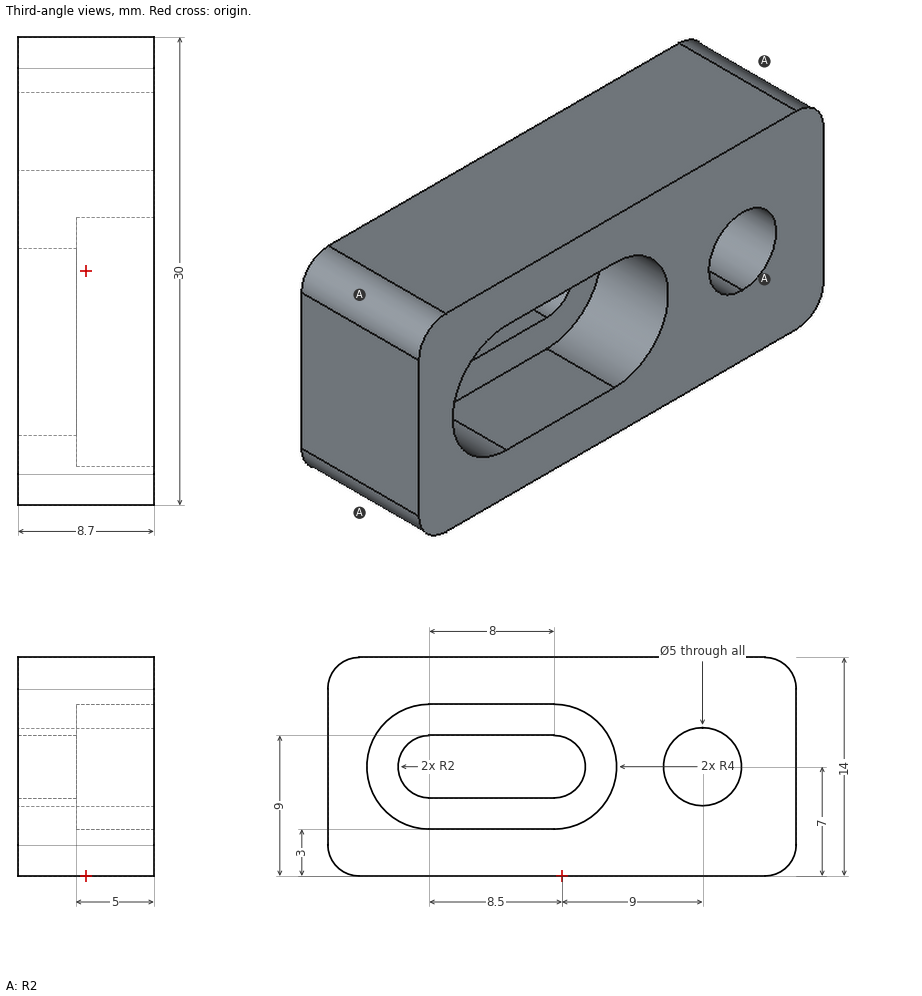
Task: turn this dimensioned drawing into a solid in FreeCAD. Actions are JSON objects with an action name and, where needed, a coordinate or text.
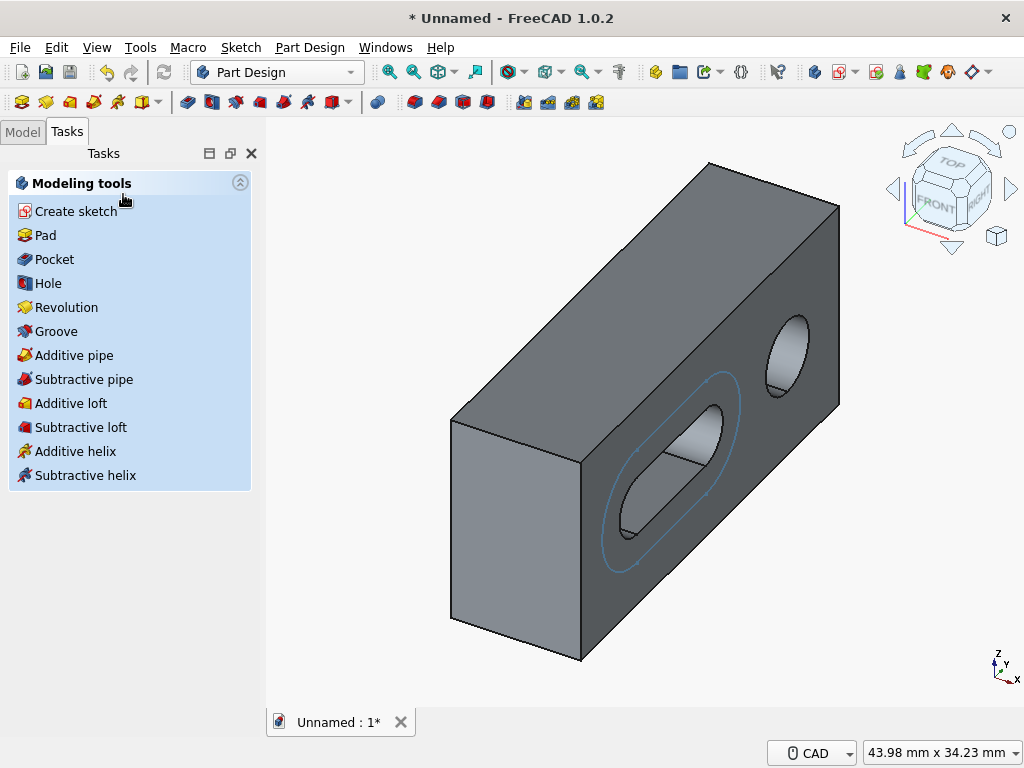
{"action": "left_click", "coordinate": [188, 102]}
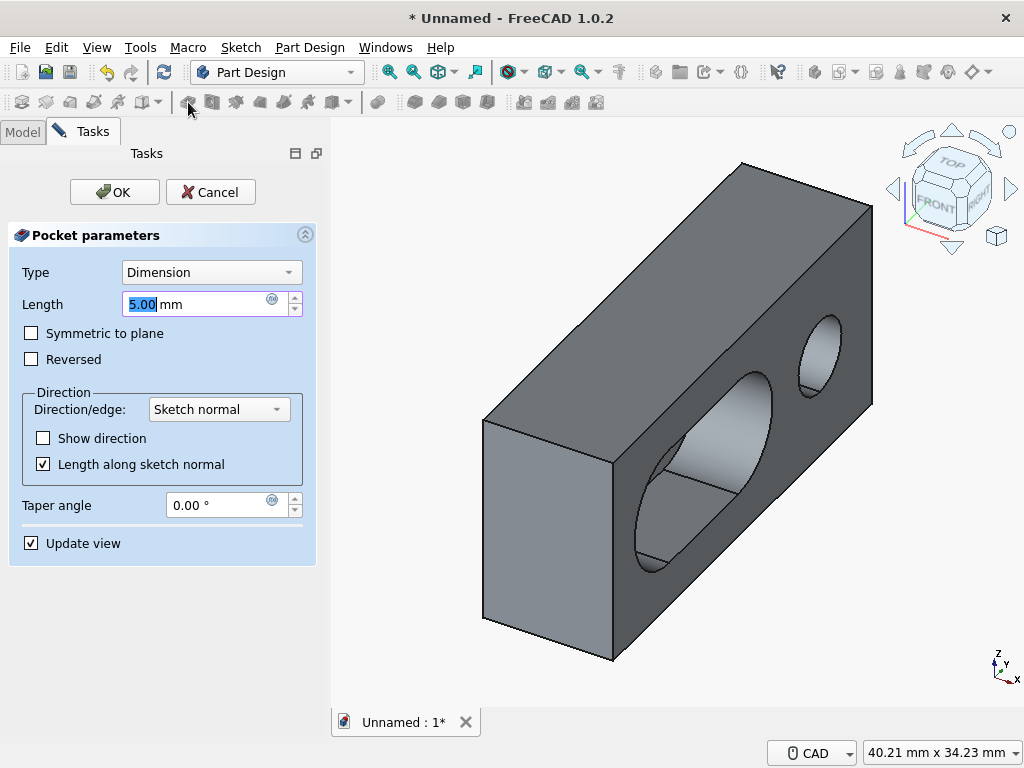
{"action": "type", "text": "5"}
{"action": "key", "text": "Tab"}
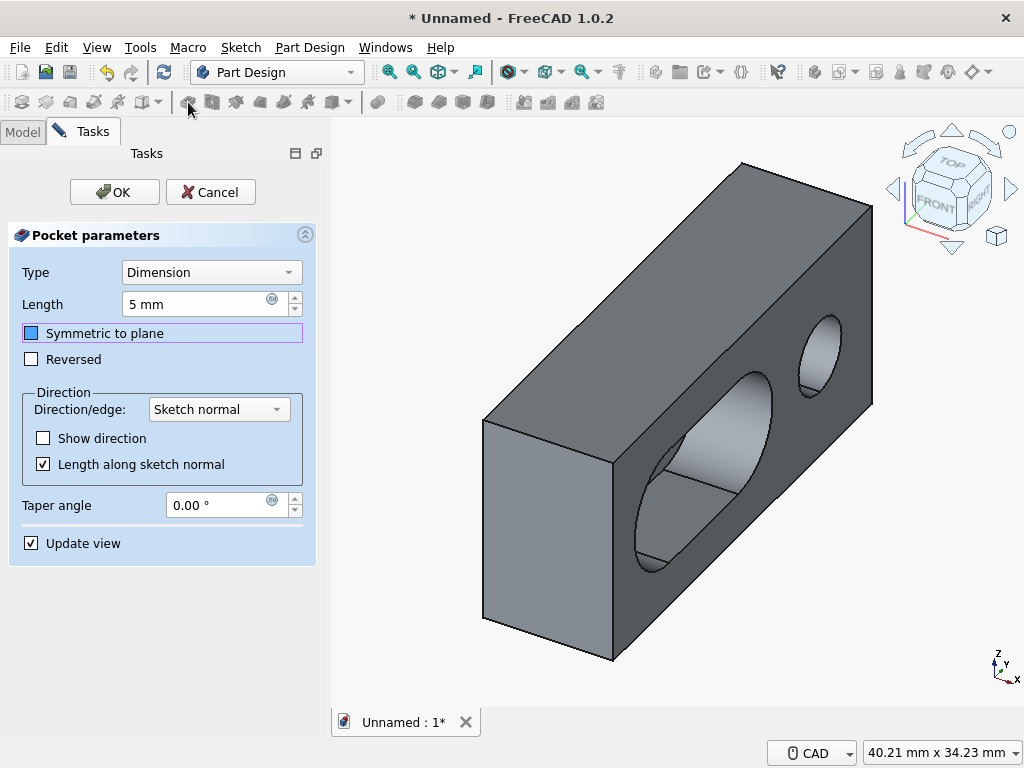
{"action": "left_click", "coordinate": [115, 192]}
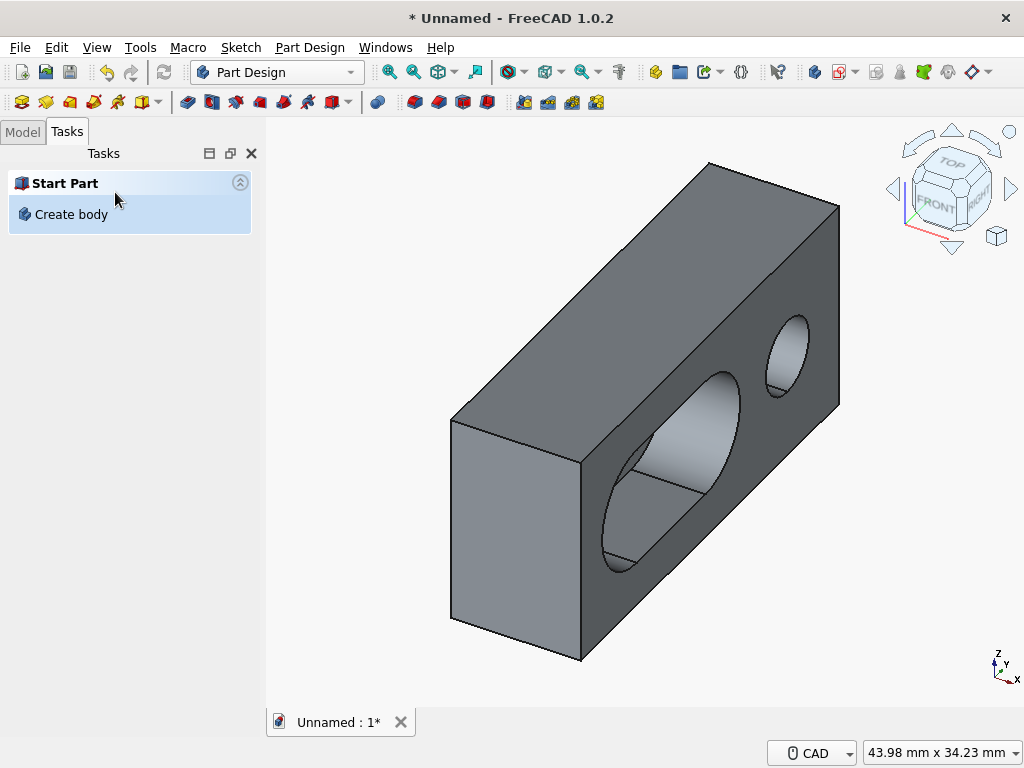
{"action": "left_click", "coordinate": [516, 441]}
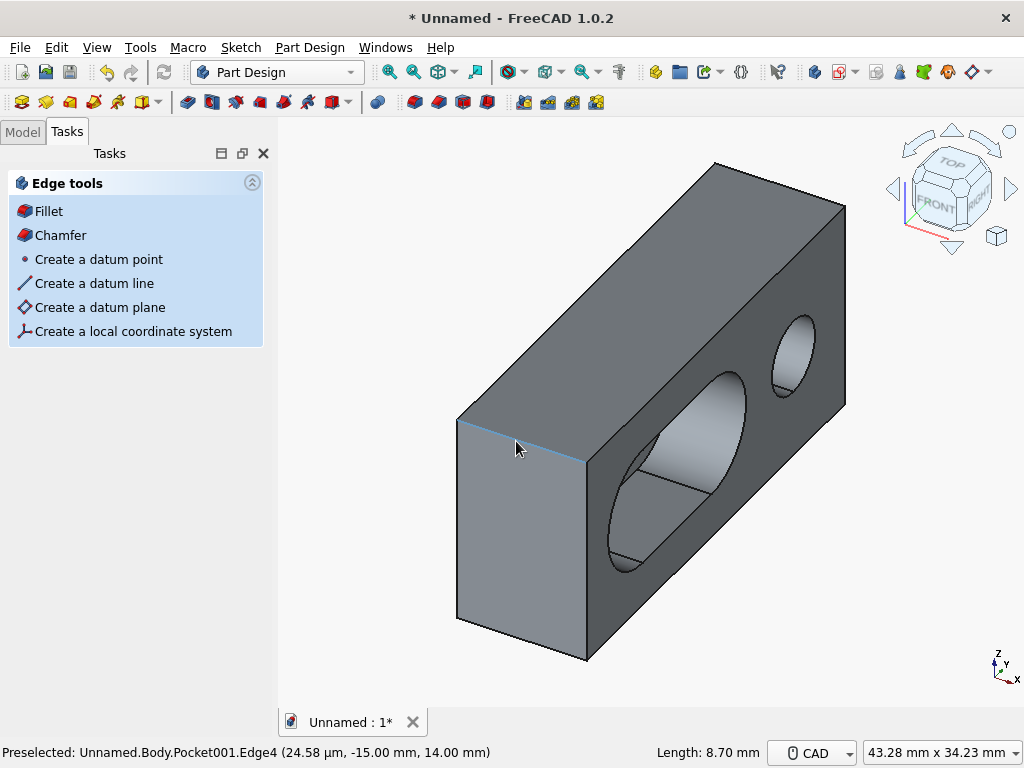
{"action": "key", "text": "0"}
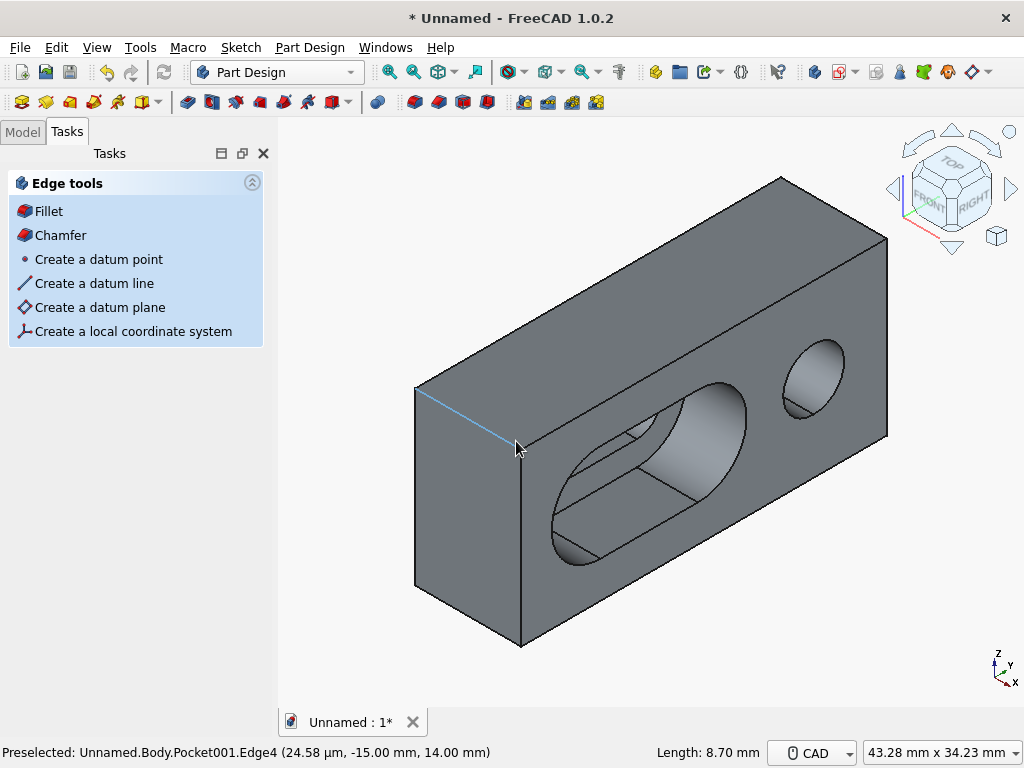
{"action": "key", "text": "2"}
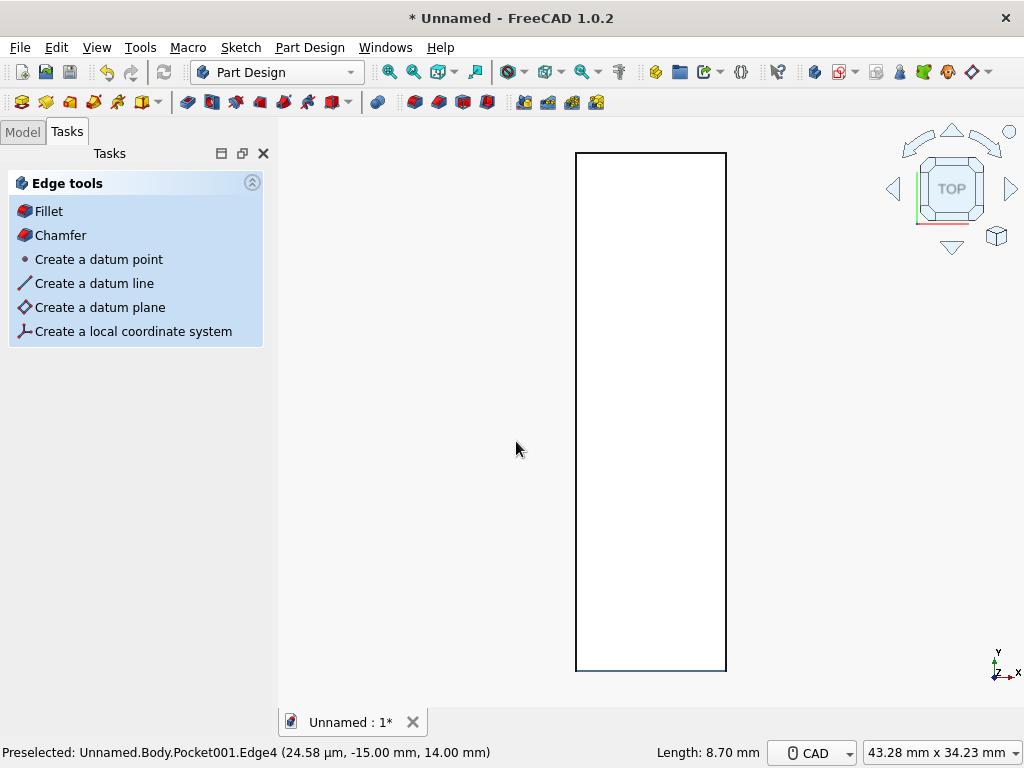
{"action": "left_click", "coordinate": [651, 152], "text": "ctrl"}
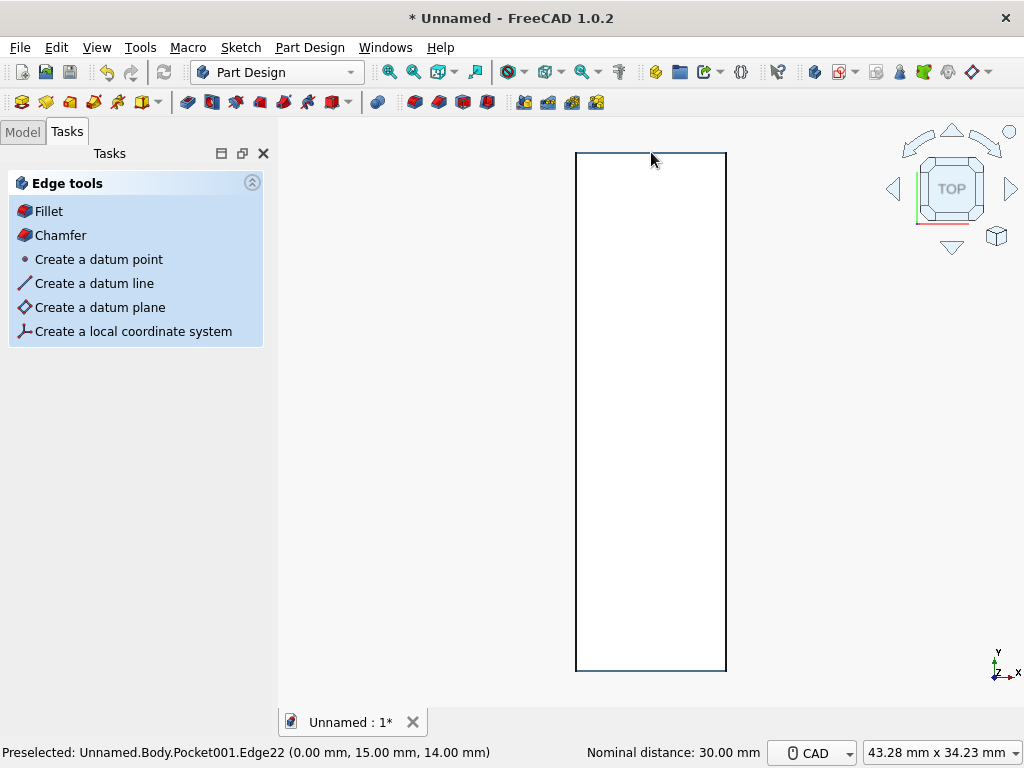
{"action": "key", "text": "1"}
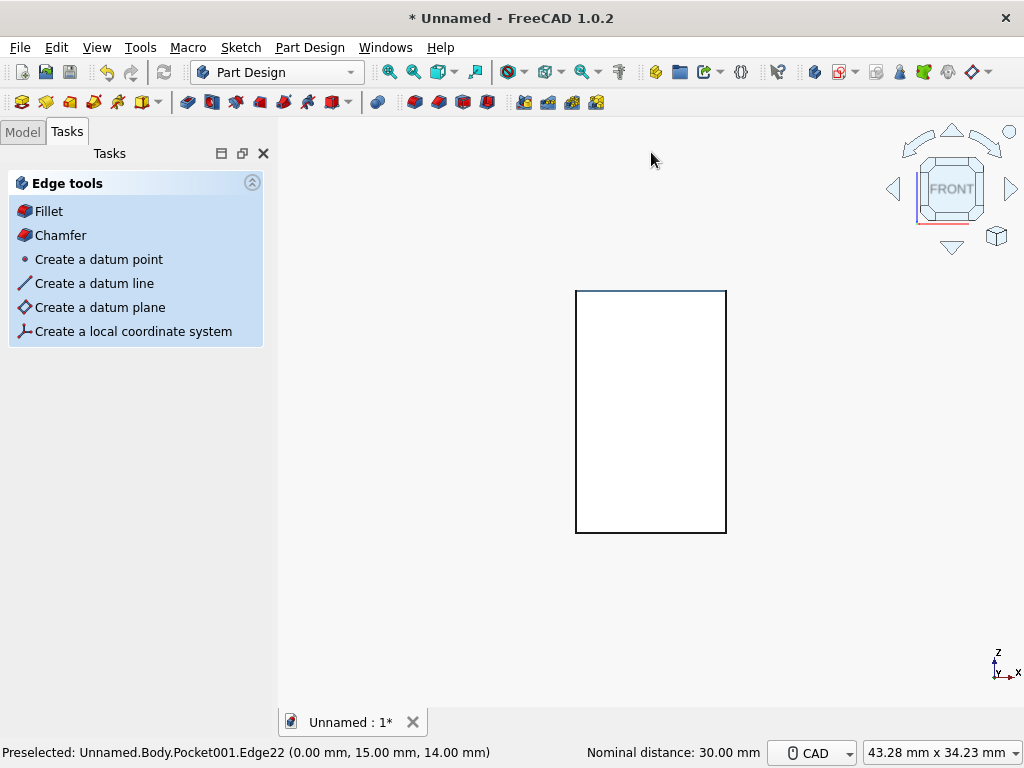
{"action": "left_click", "coordinate": [390, 72]}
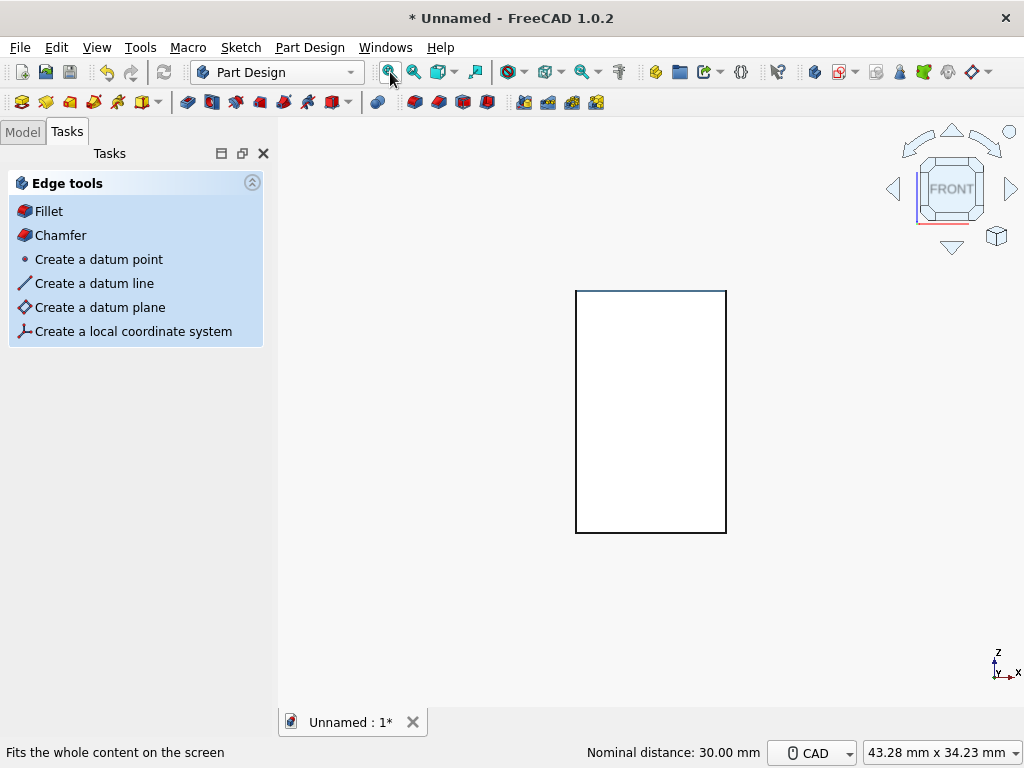
{"action": "left_click", "coordinate": [651, 532], "text": "ctrl"}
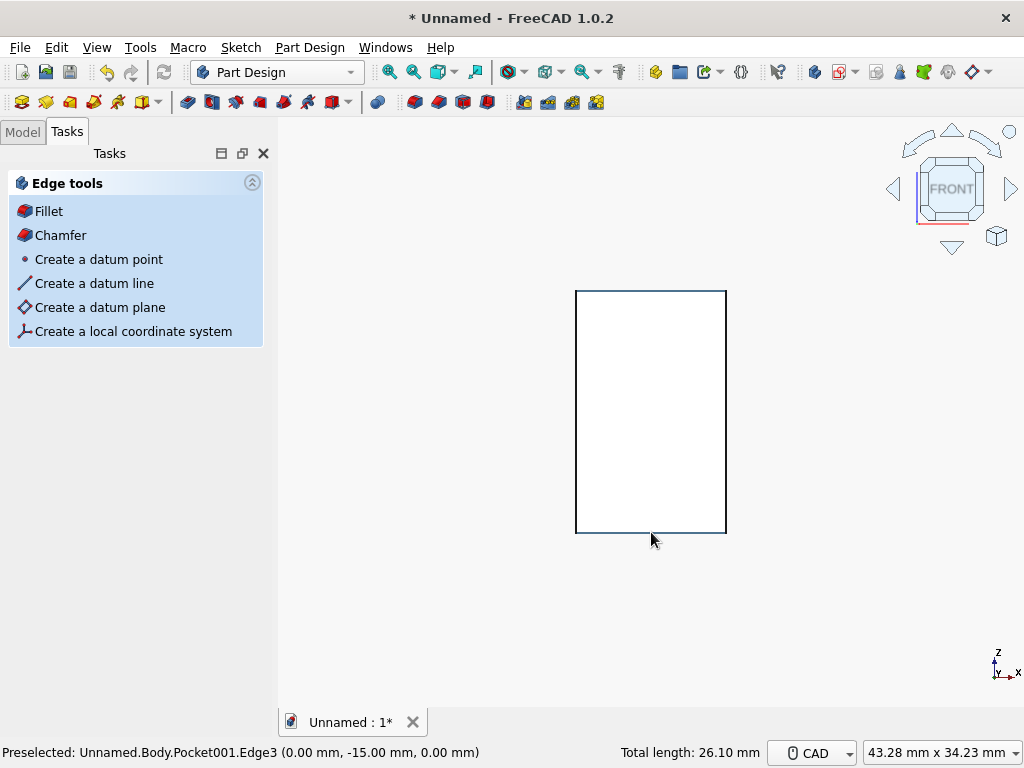
{"action": "key", "text": "3"}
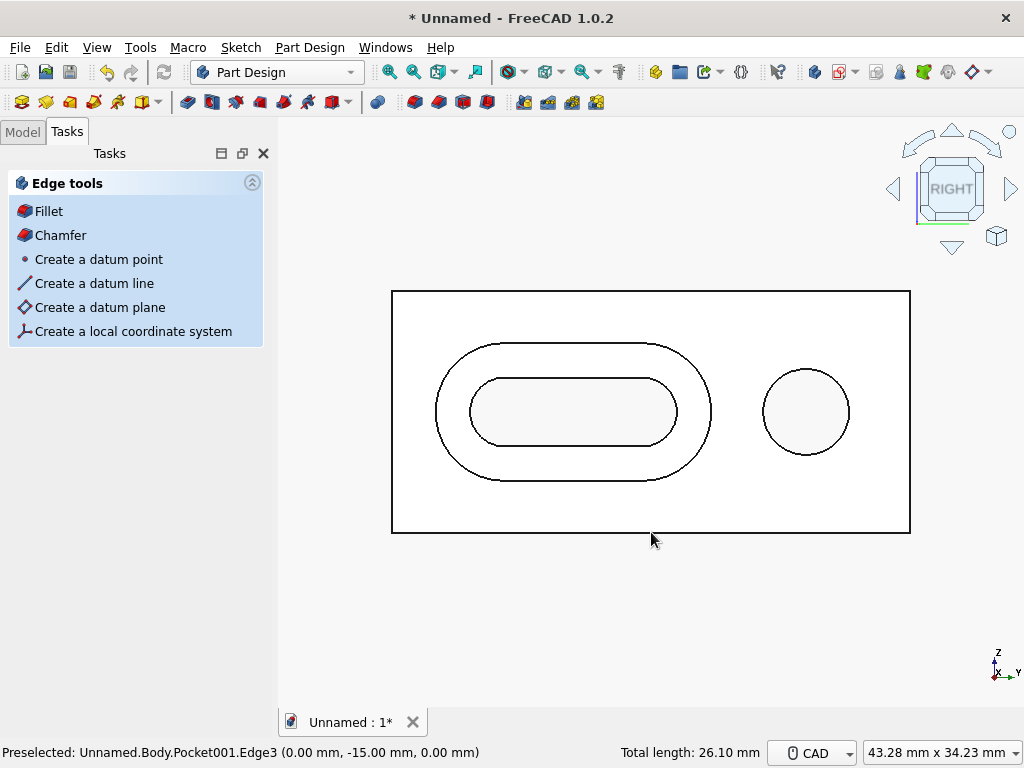
{"action": "key", "text": "5"}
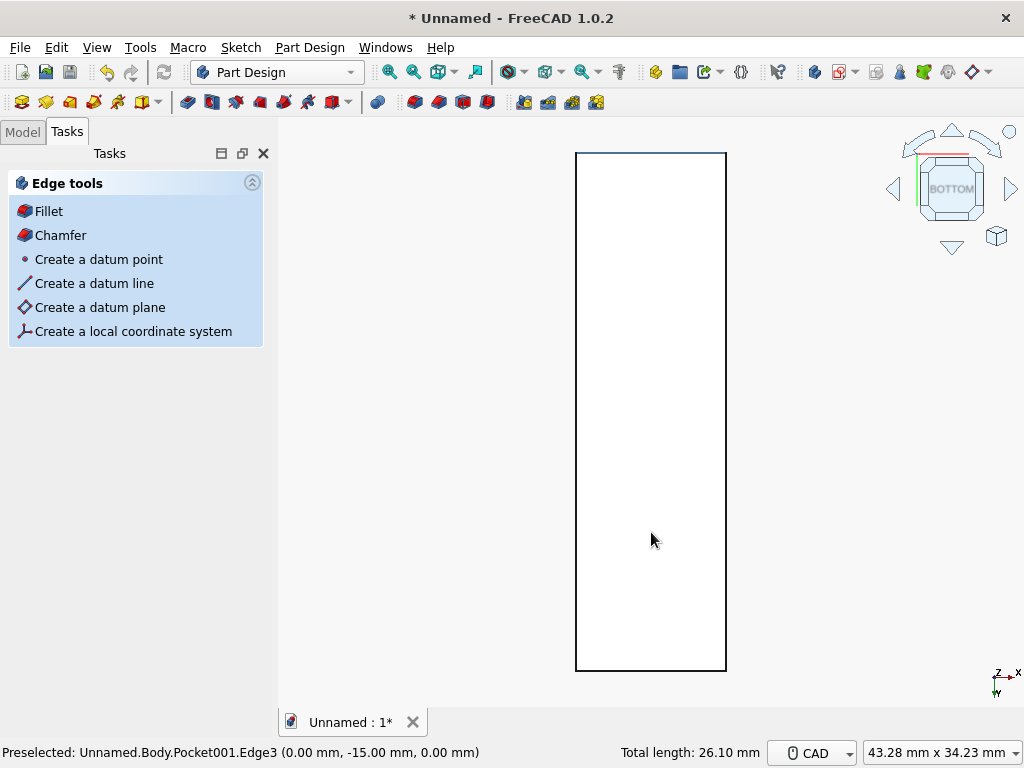
{"action": "left_click", "coordinate": [651, 670], "text": "ctrl"}